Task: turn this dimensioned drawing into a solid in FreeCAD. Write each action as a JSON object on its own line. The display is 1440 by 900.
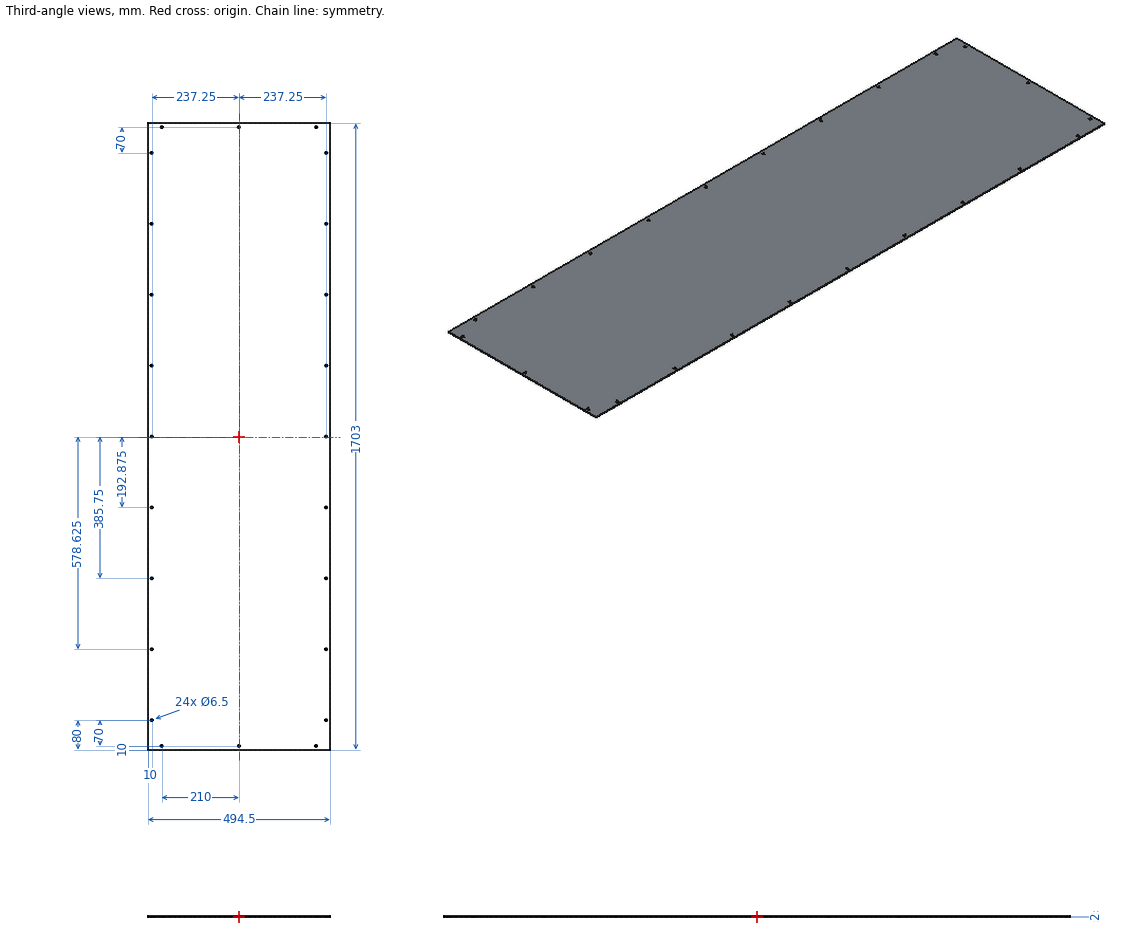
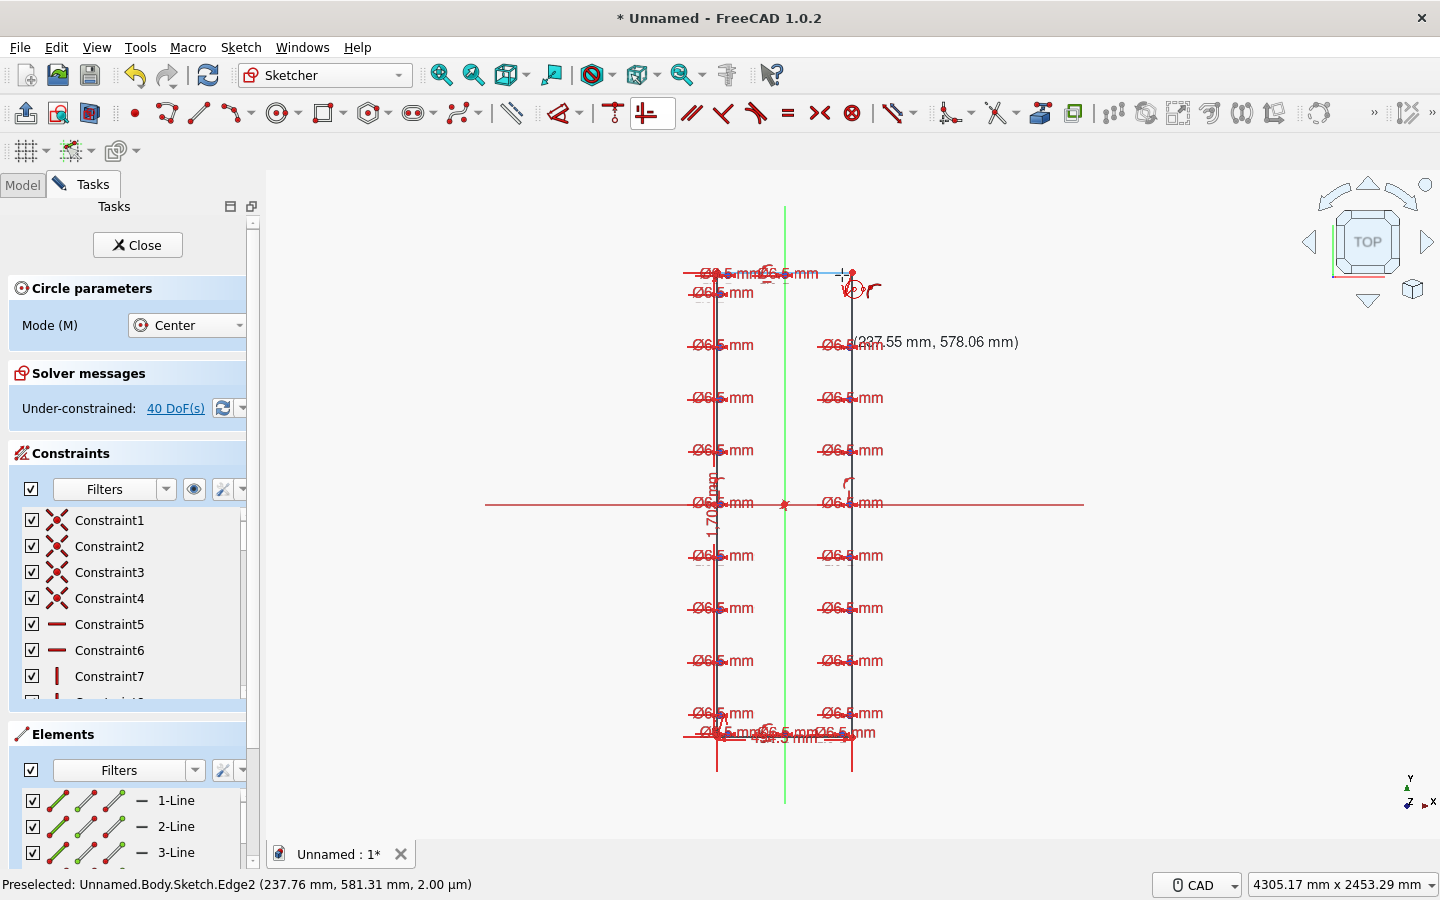
{"action": "scroll", "coordinate": [842, 275], "scroll_direction": "up", "scroll_amount": 9}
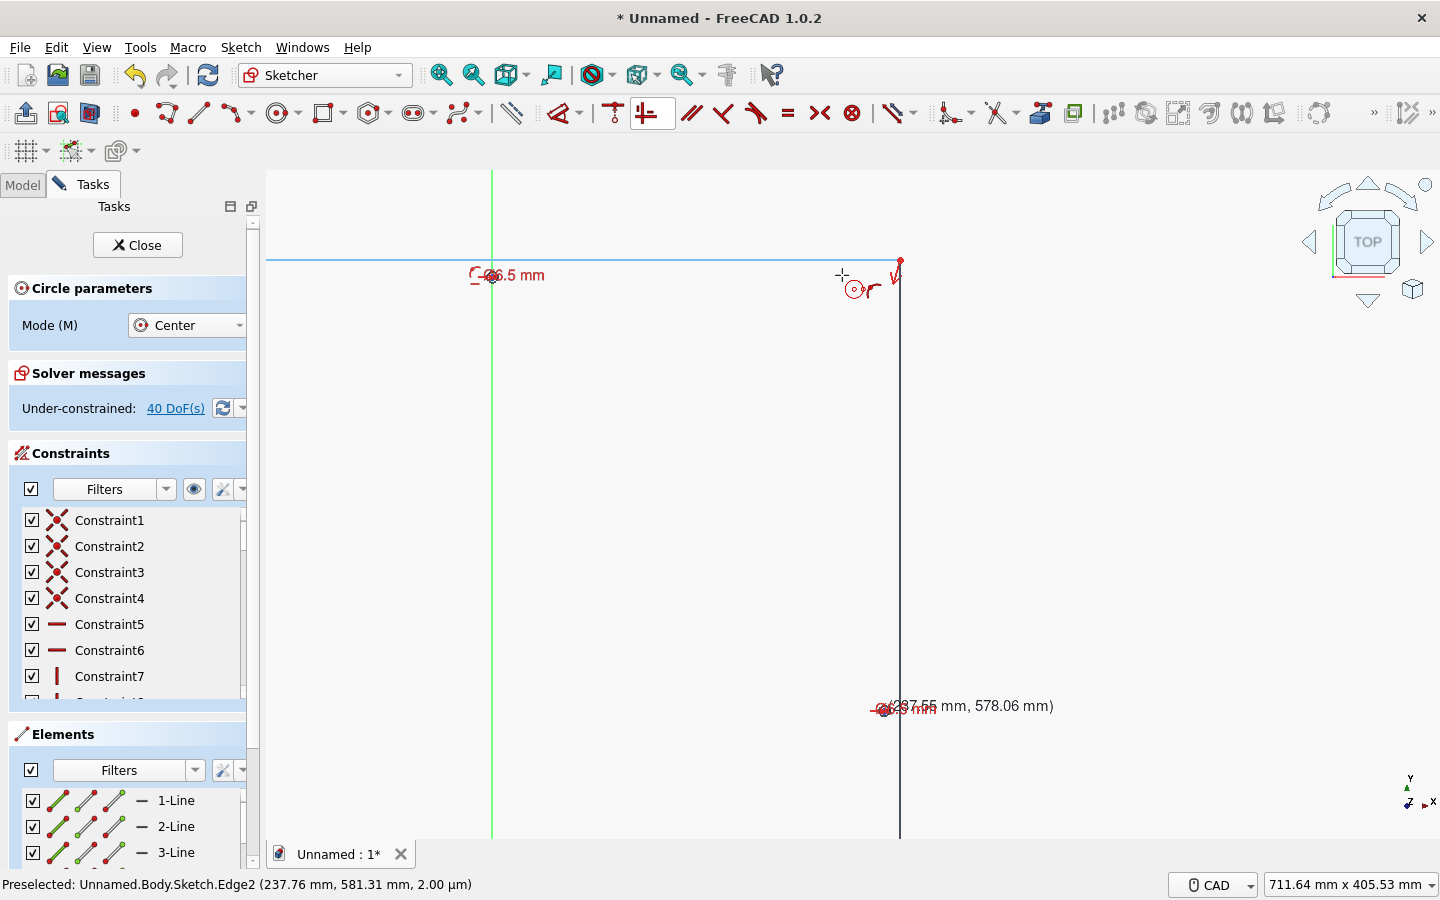
{"action": "left_click", "coordinate": [839, 277]}
{"action": "mouse_move", "coordinate": [843, 280]}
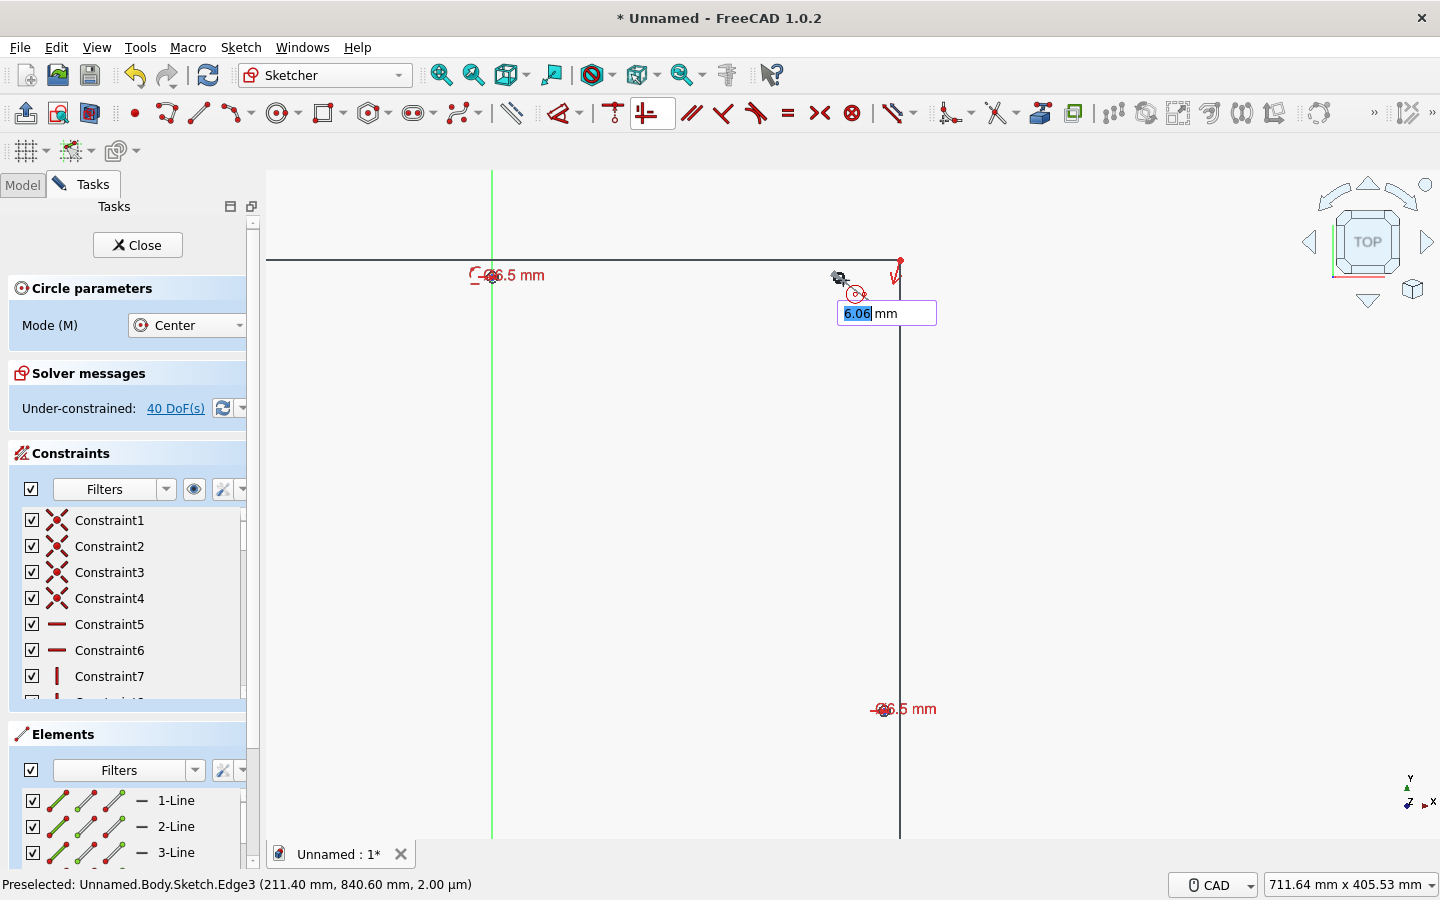
{"action": "type", "text": "6.5"}
{"action": "key", "text": "Return"}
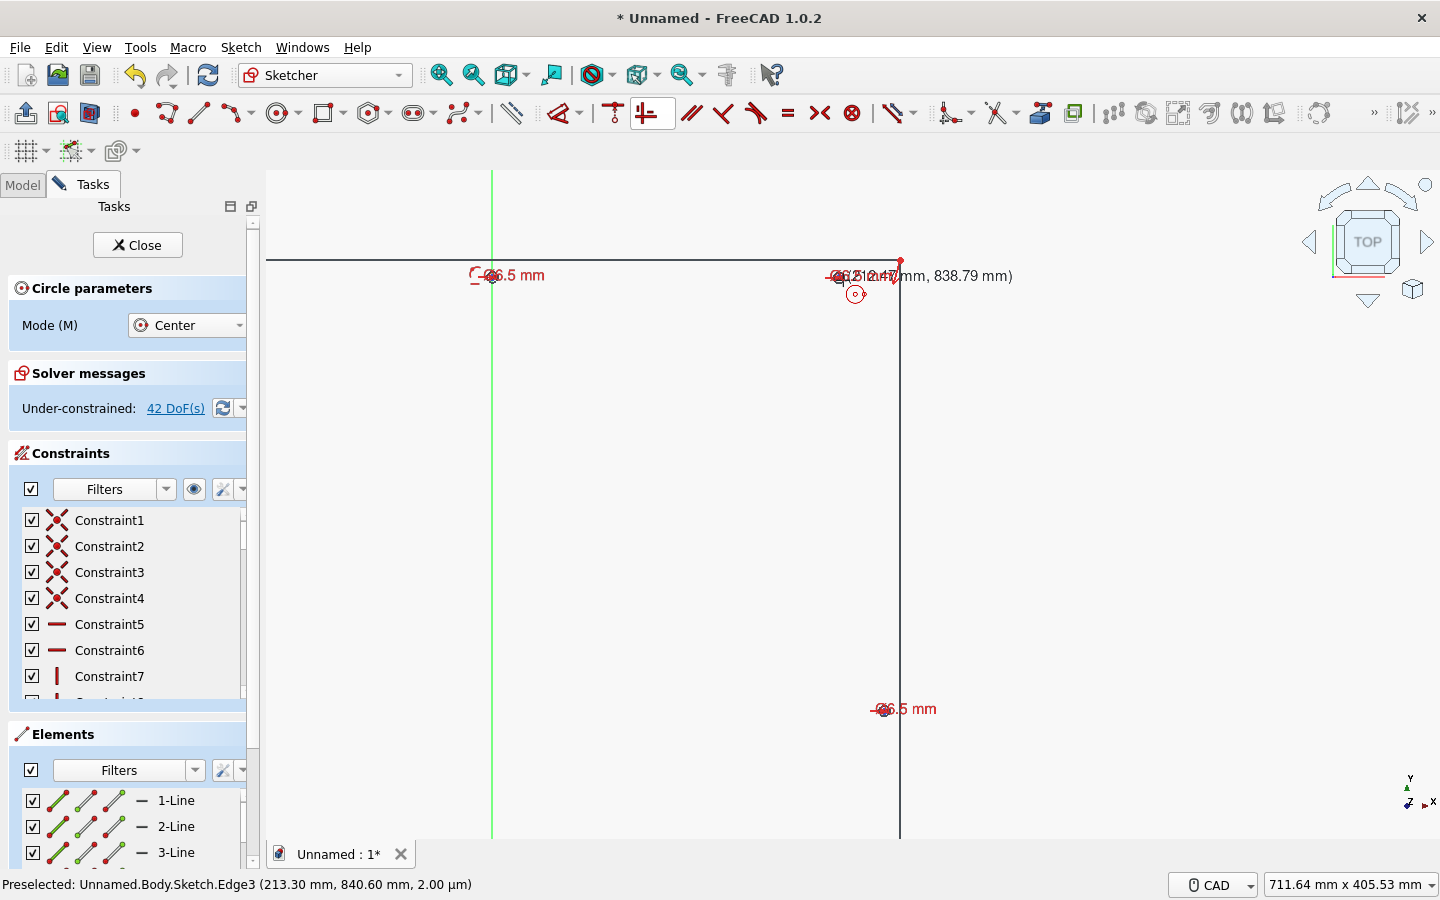
{"action": "scroll", "coordinate": [884, 392], "scroll_direction": "up", "scroll_amount": 8}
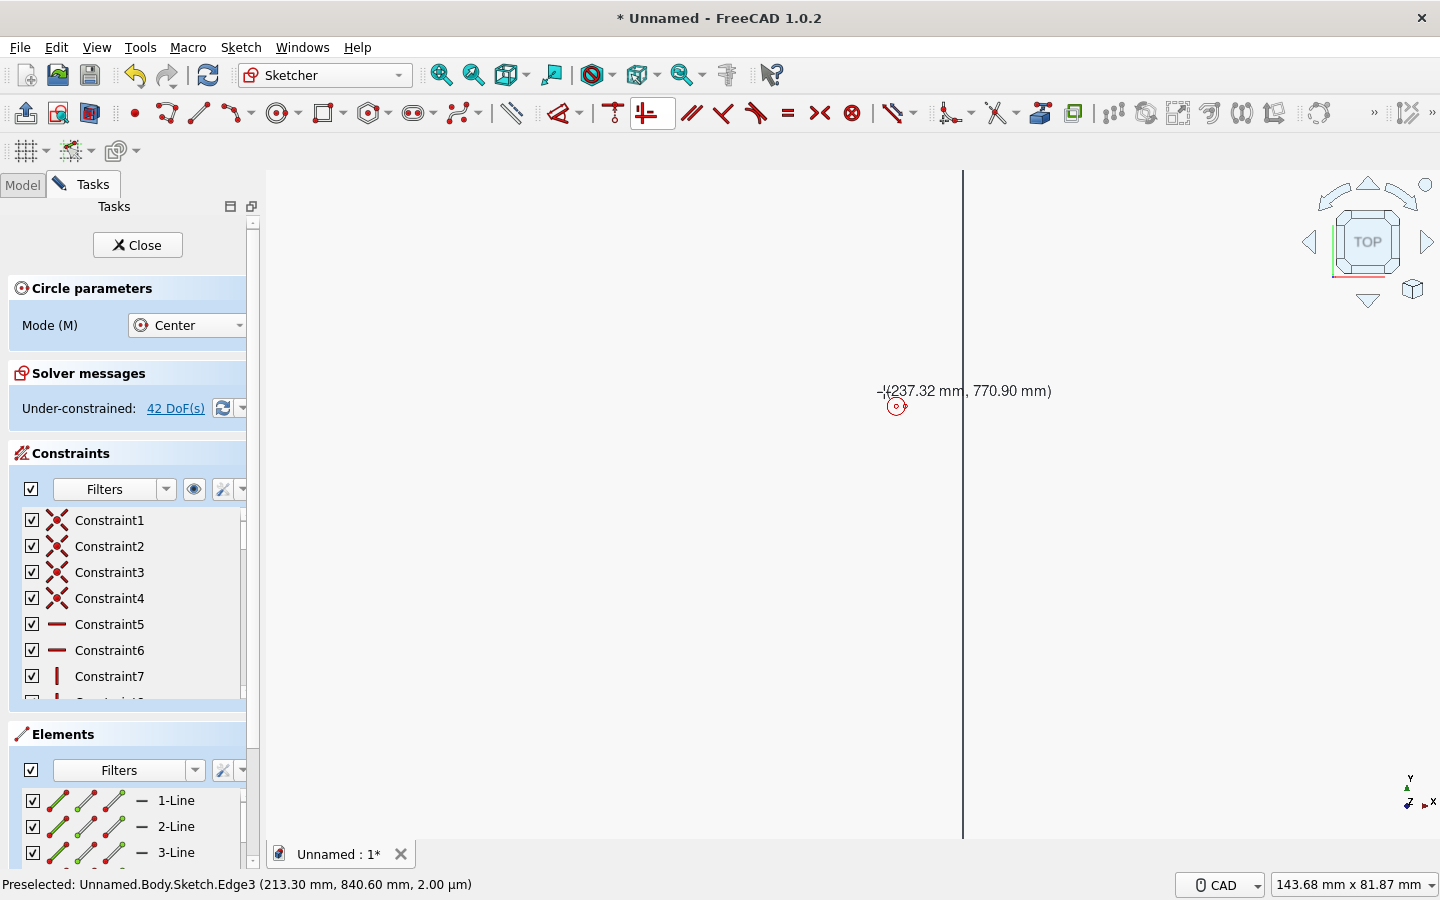
{"action": "scroll", "coordinate": [848, 291], "scroll_direction": "down", "scroll_amount": 17}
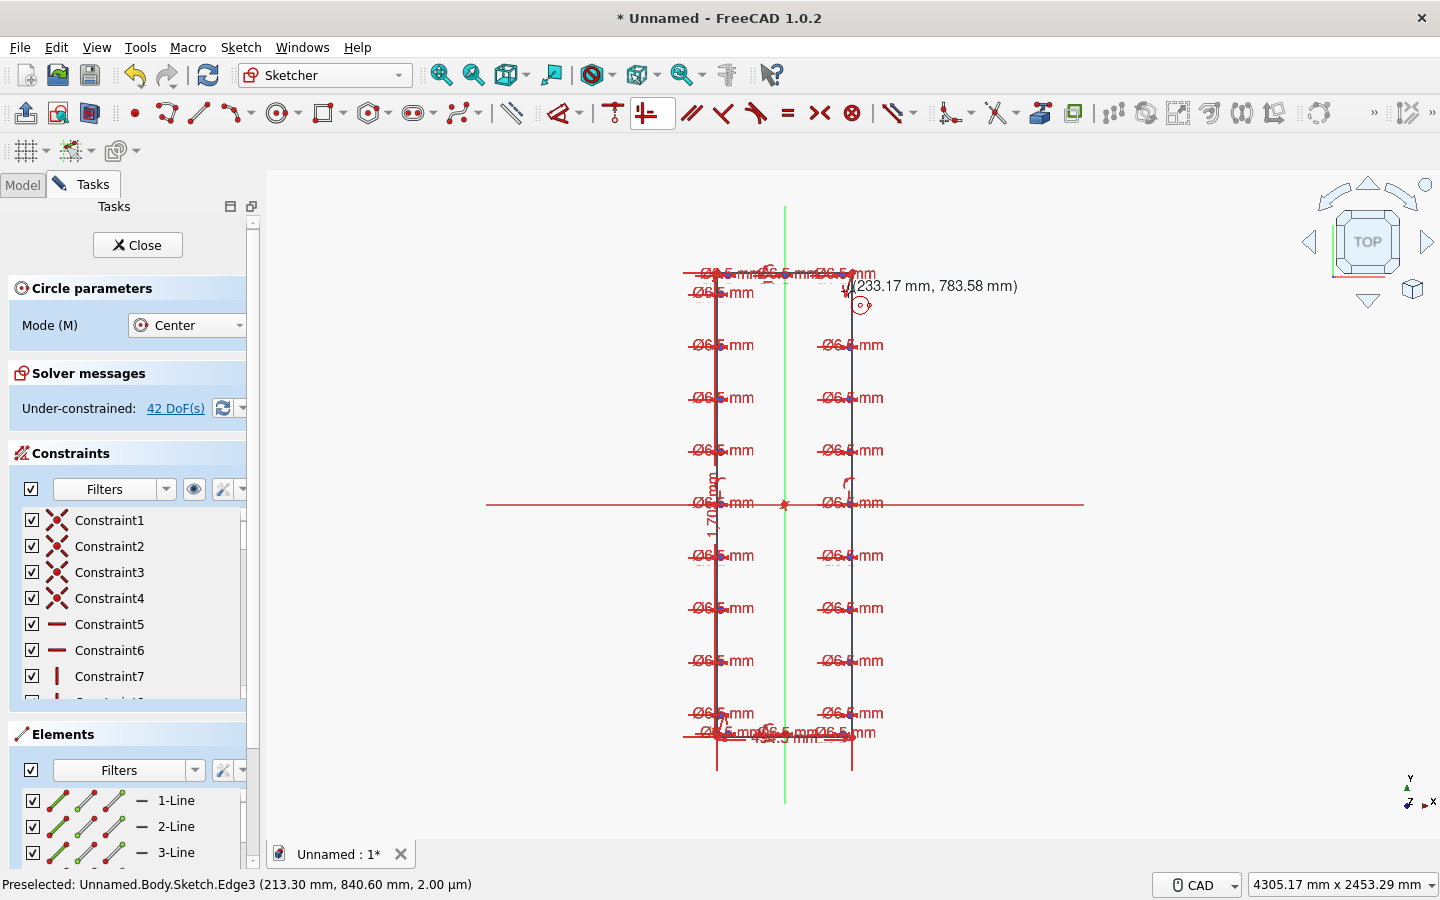
{"action": "scroll", "coordinate": [850, 295], "scroll_direction": "up", "scroll_amount": 9}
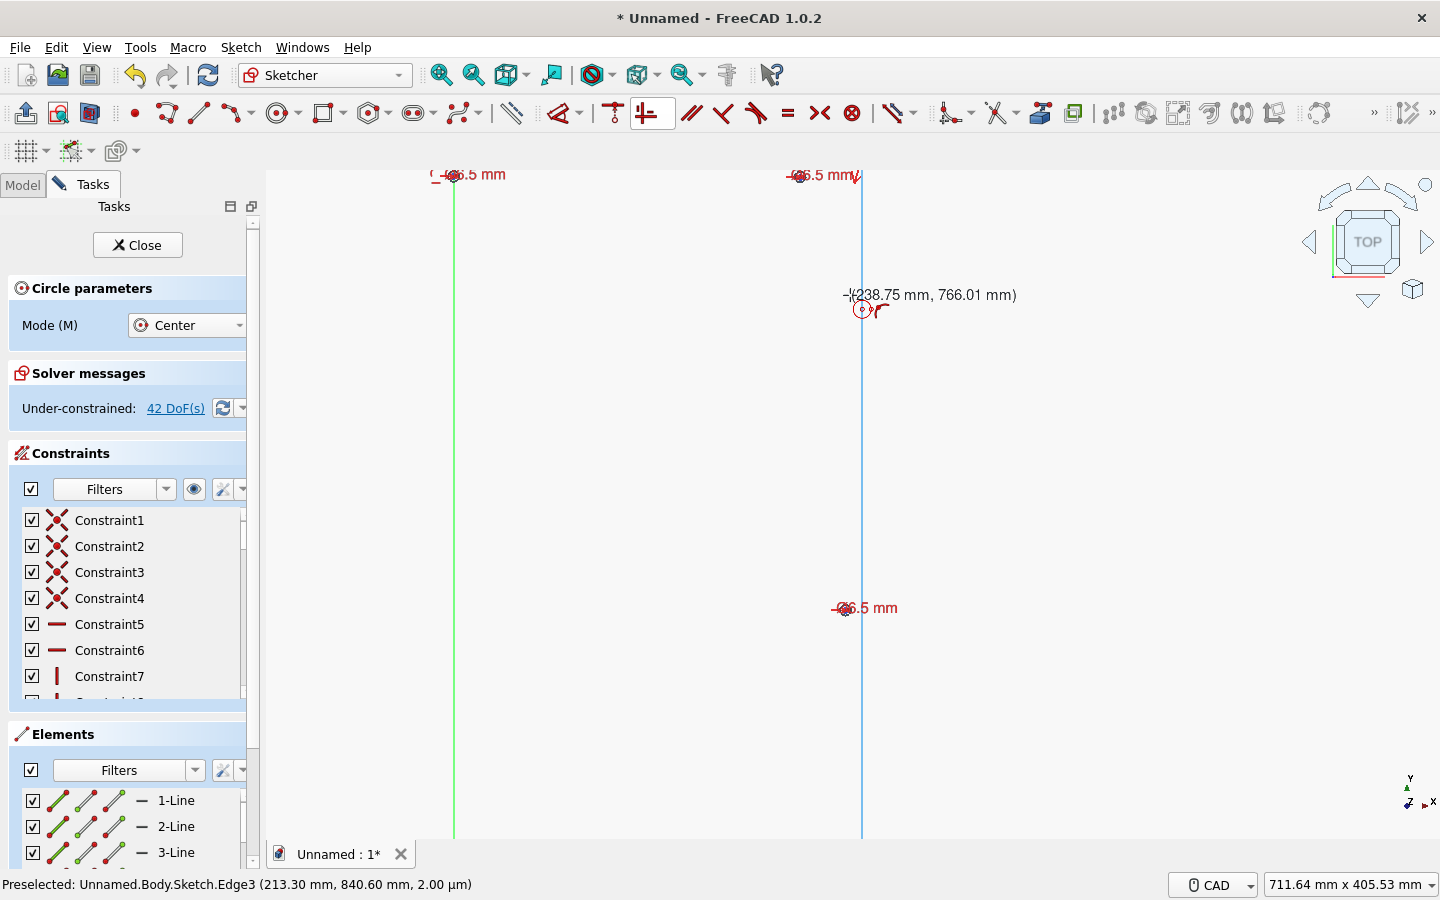
{"action": "left_click", "coordinate": [845, 291]}
{"action": "mouse_move", "coordinate": [841, 287]}